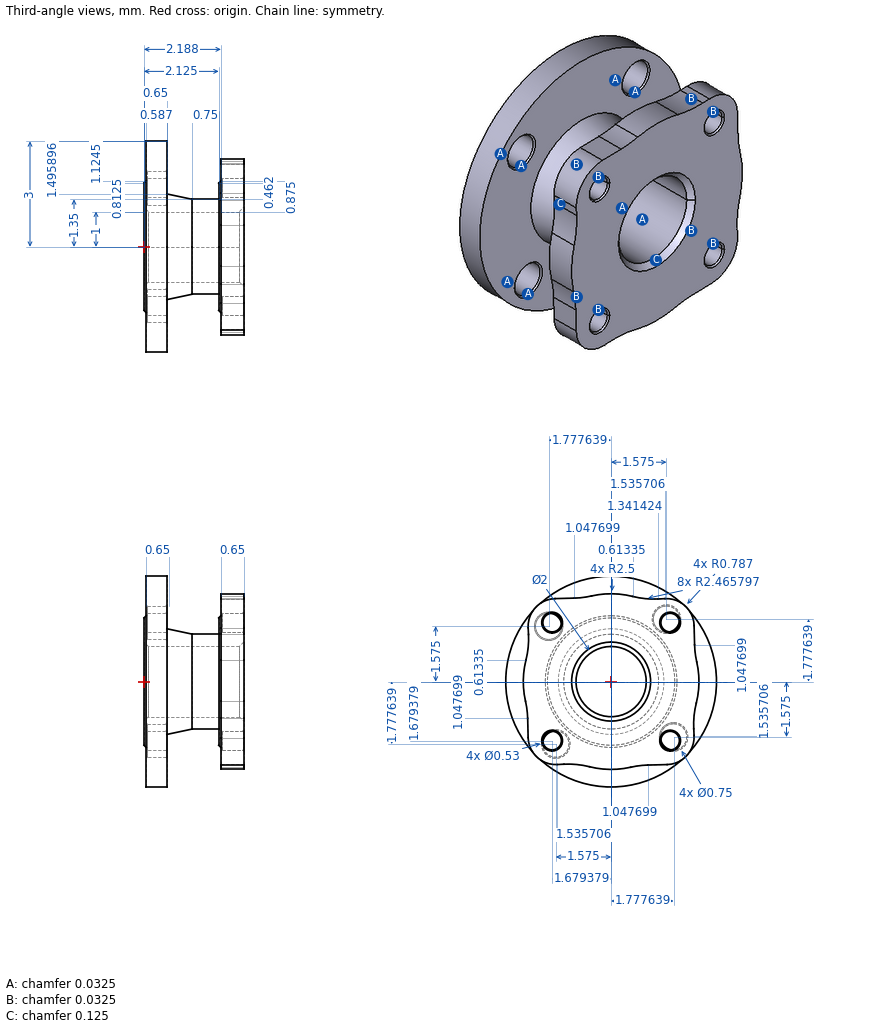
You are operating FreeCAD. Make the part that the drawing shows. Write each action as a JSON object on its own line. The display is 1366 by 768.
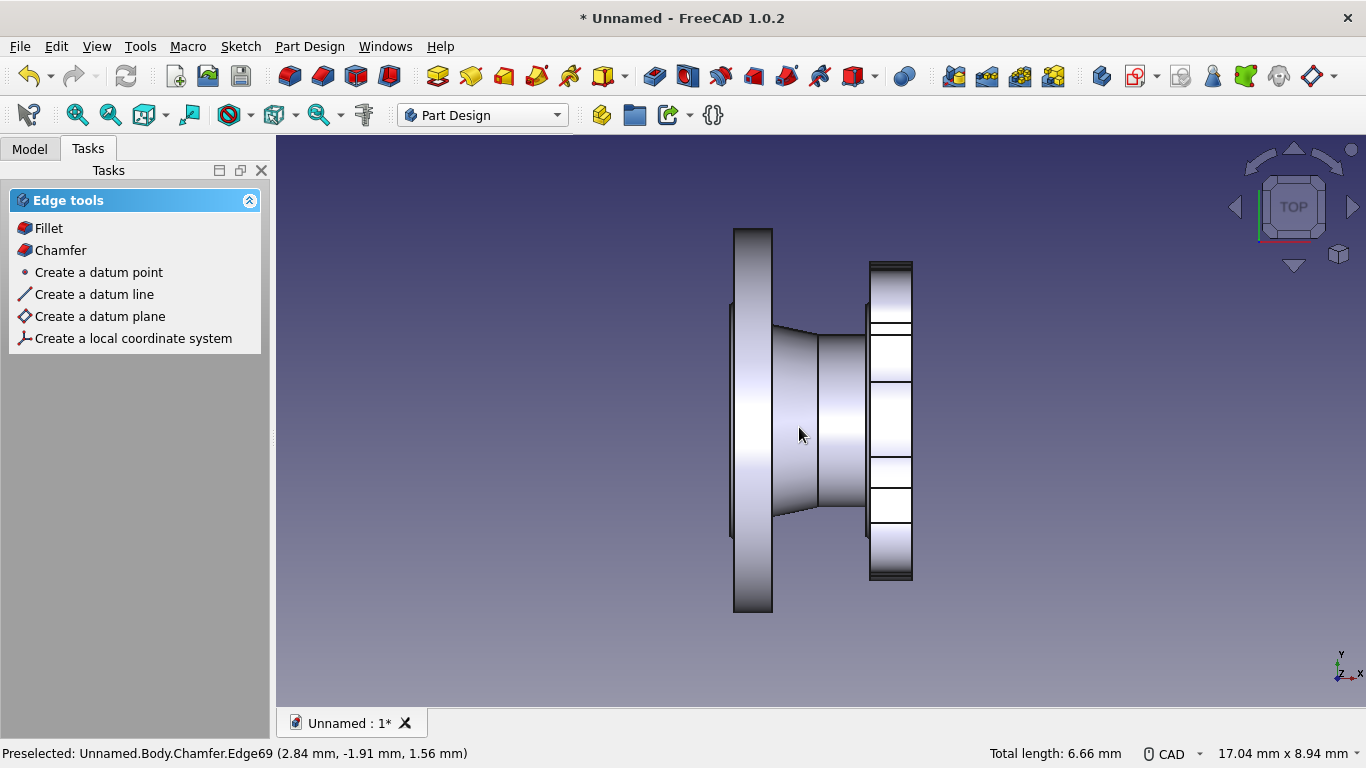
{"action": "key", "text": "0"}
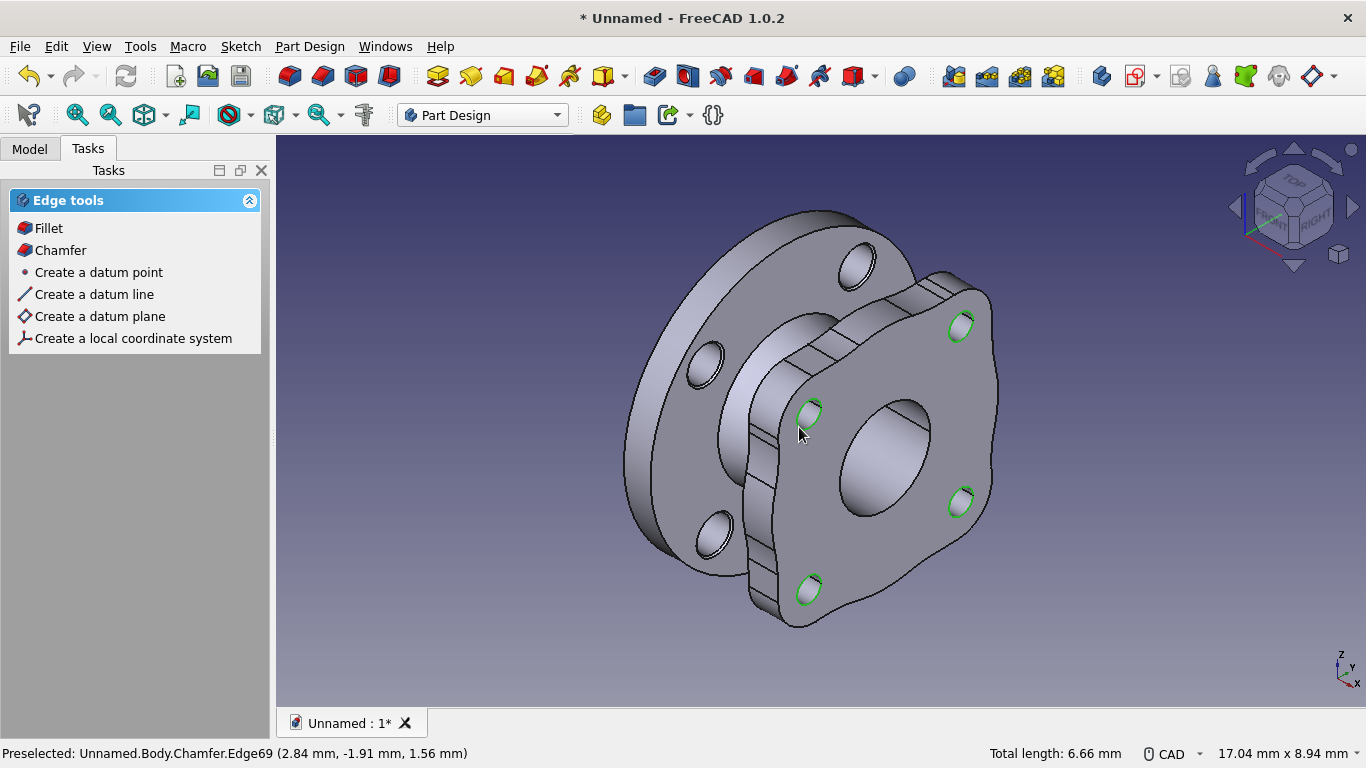
{"action": "key", "text": "1"}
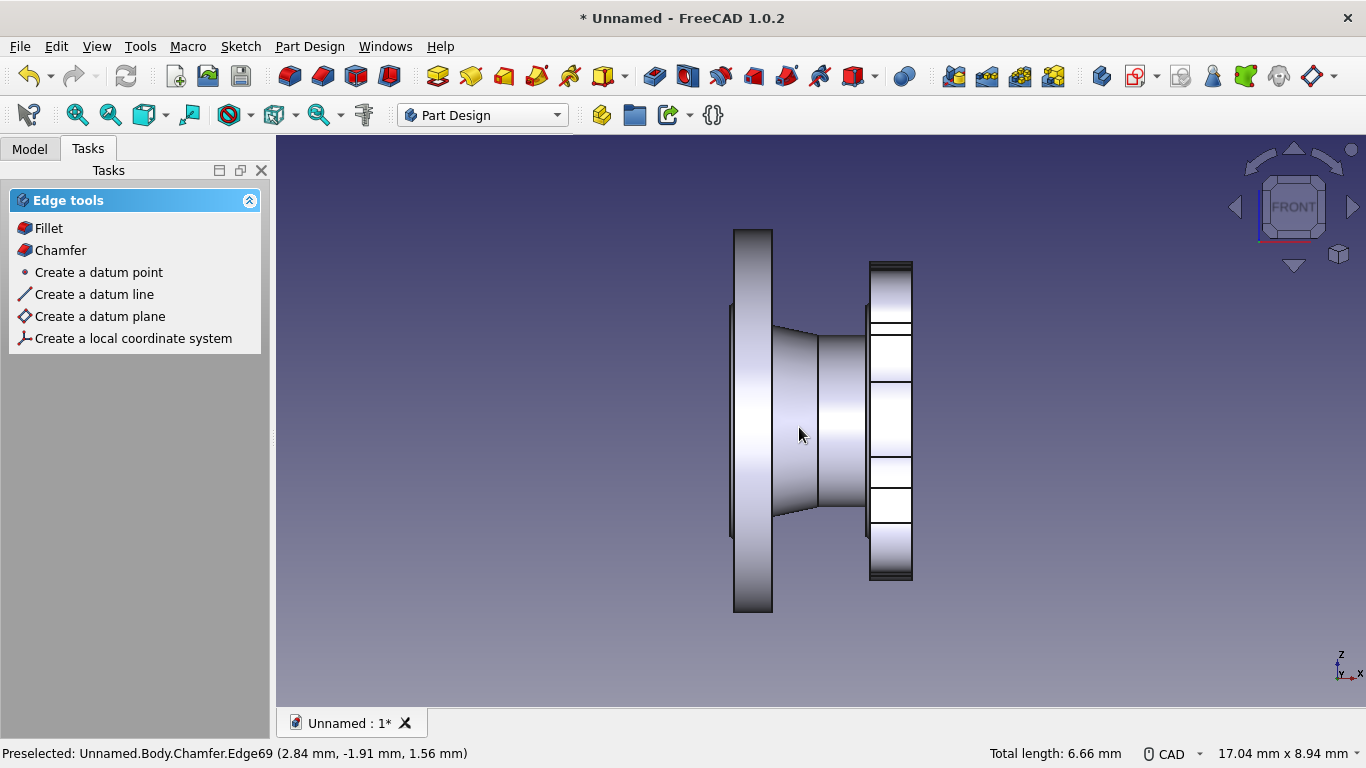
{"action": "key", "text": "3"}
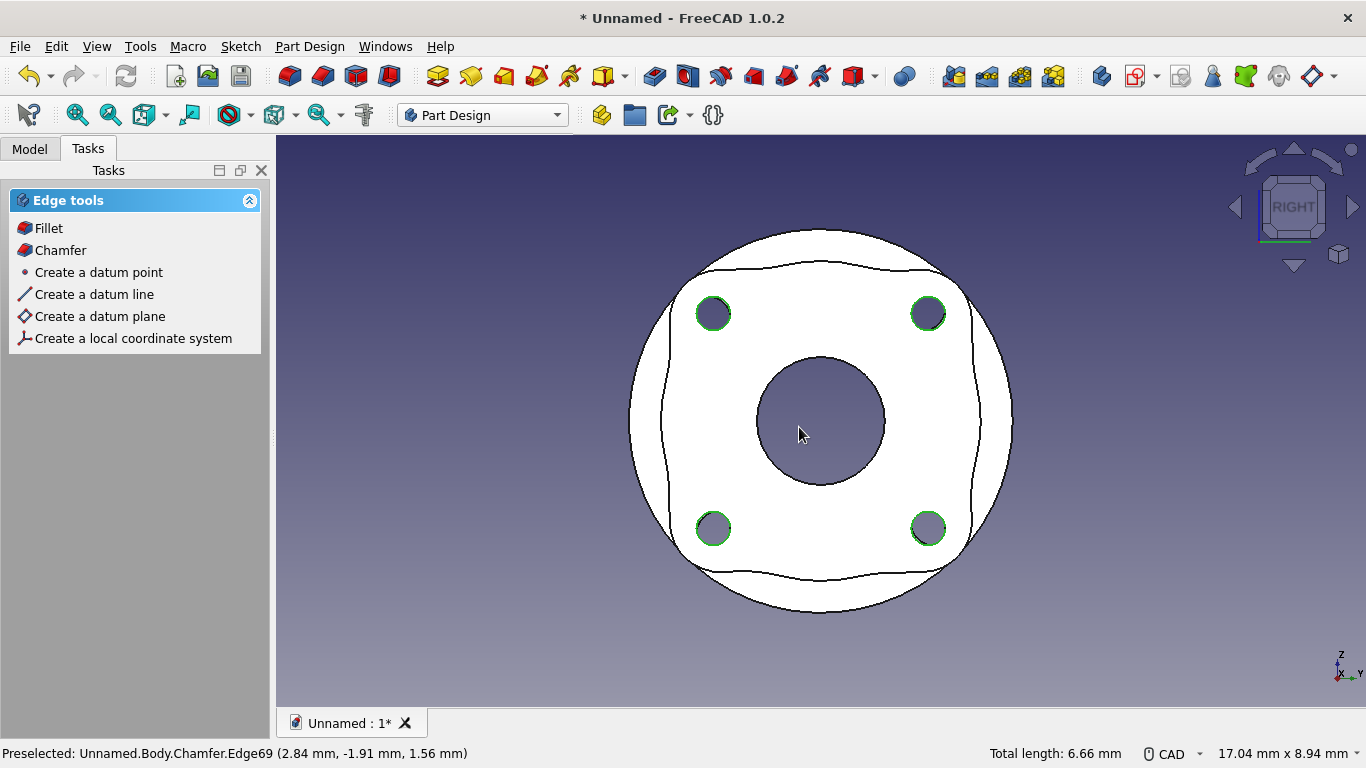
{"action": "key", "text": "5"}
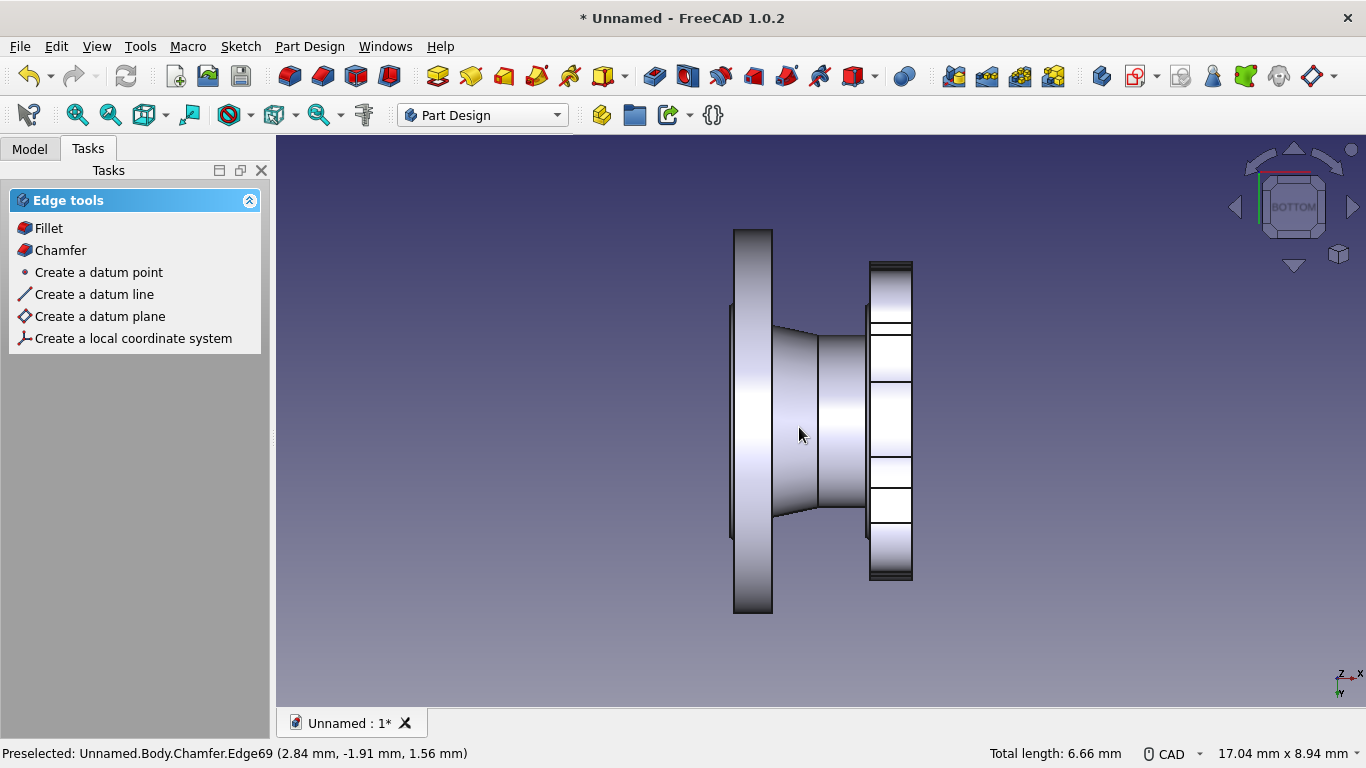
{"action": "key", "text": "4"}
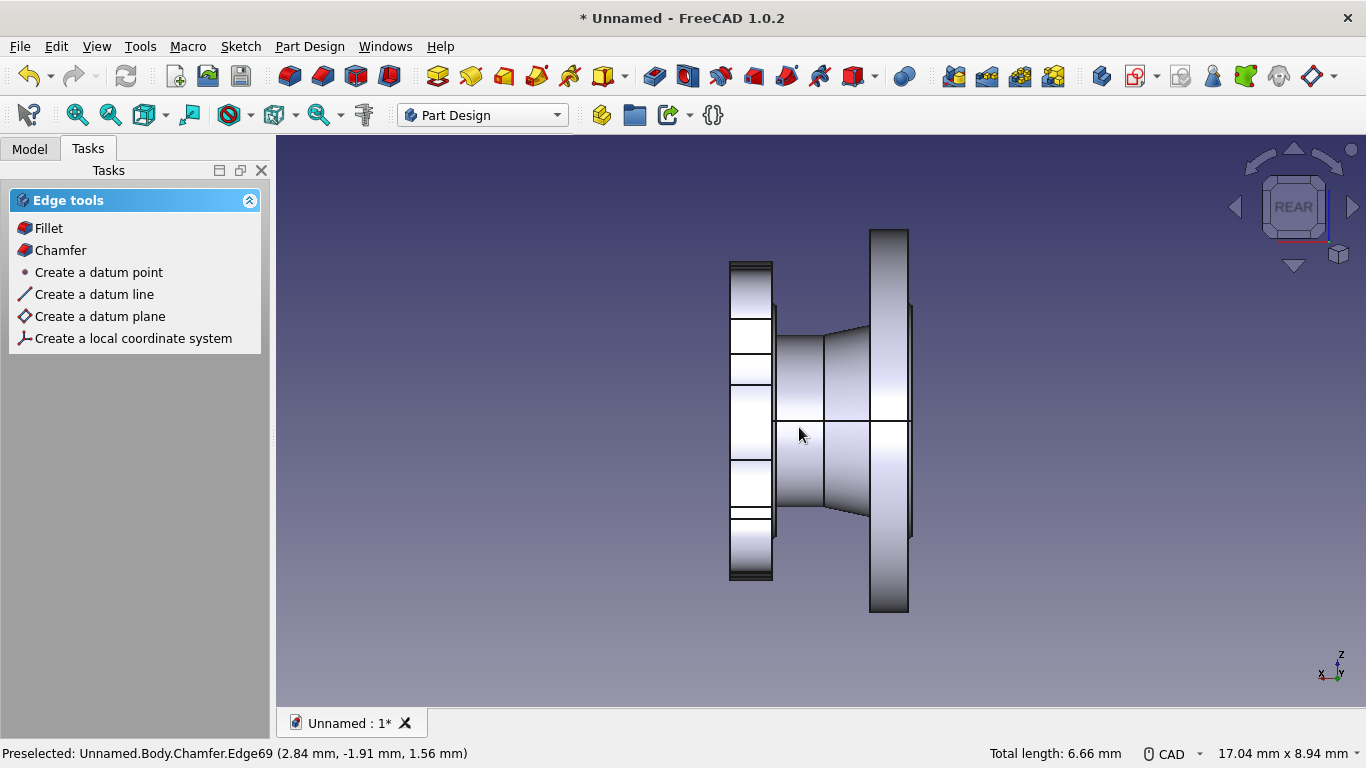
{"action": "key", "text": "6"}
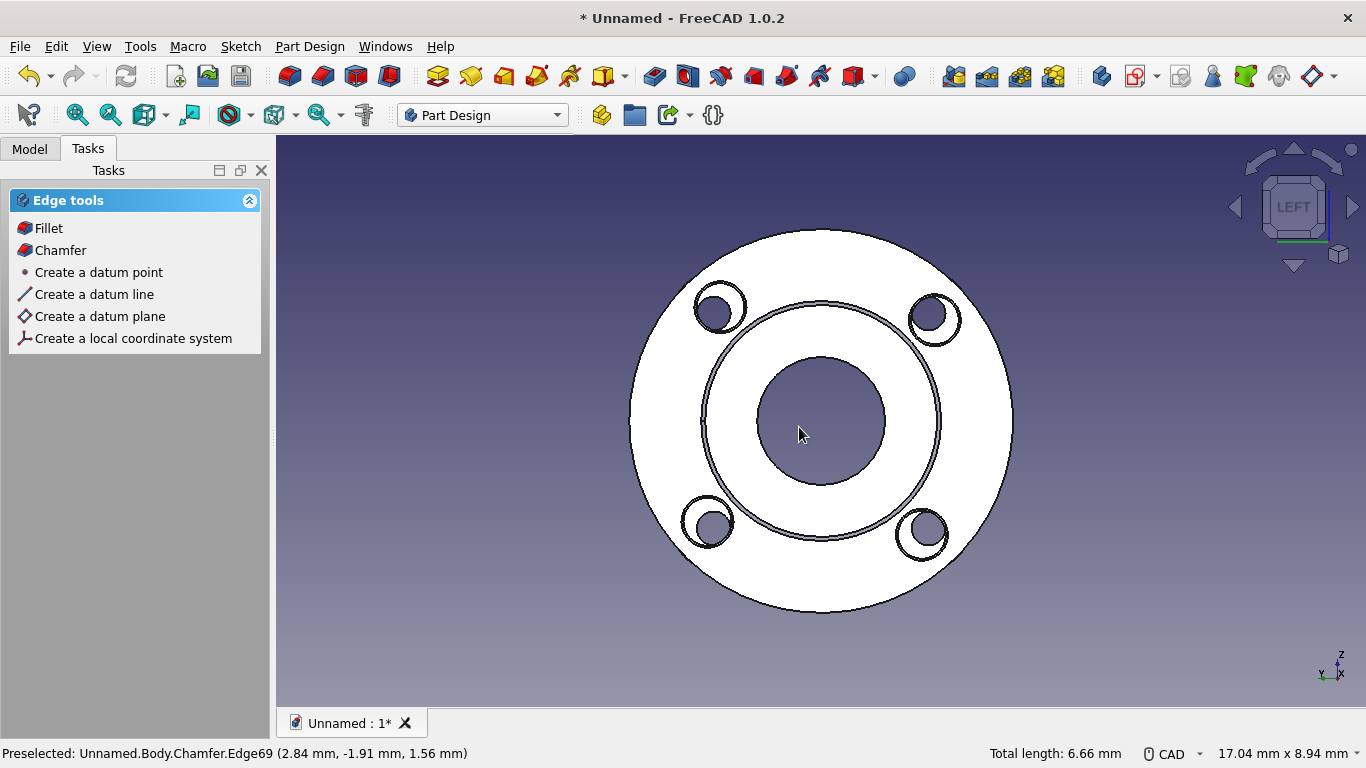
{"action": "left_click", "coordinate": [731, 313], "text": "ctrl"}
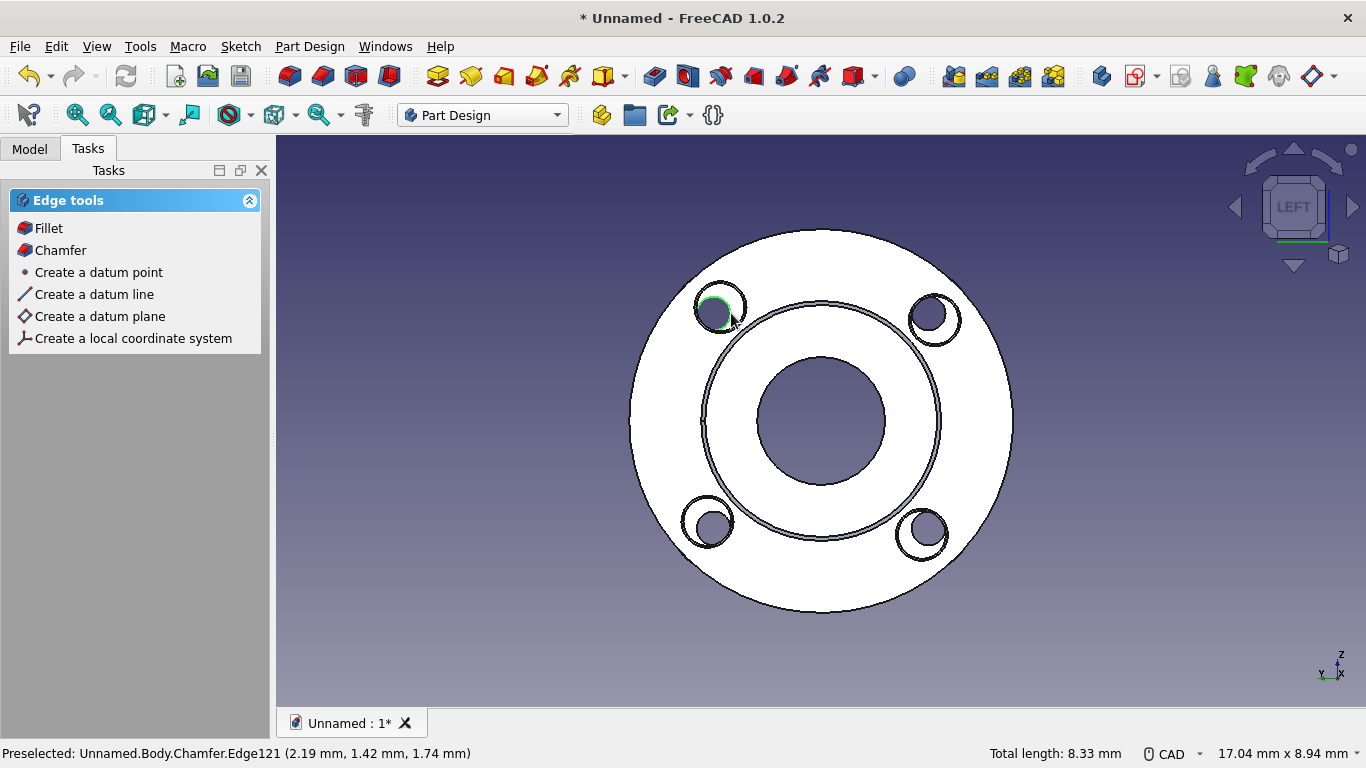
{"action": "left_click", "coordinate": [719, 511], "text": "ctrl"}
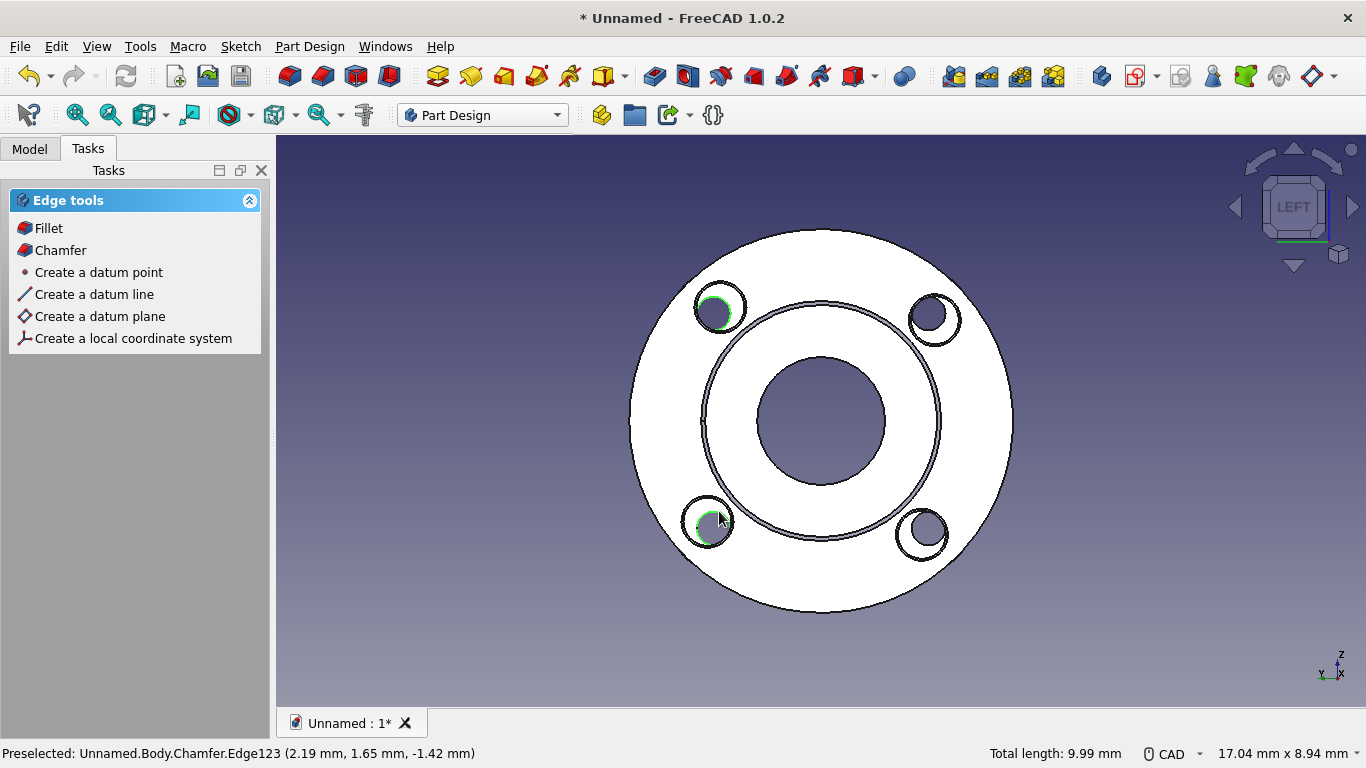
{"action": "left_click", "coordinate": [934, 544], "text": "ctrl"}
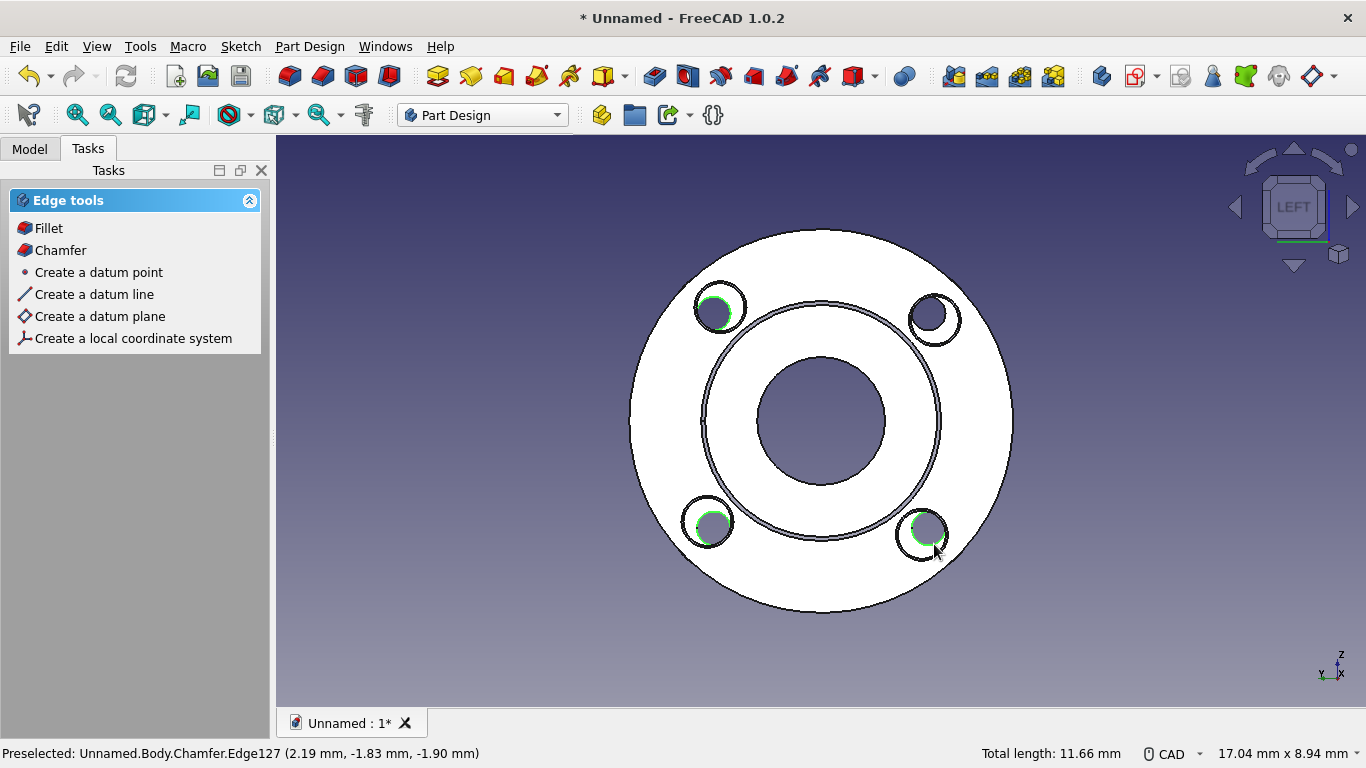
{"action": "left_click", "coordinate": [946, 313], "text": "ctrl"}